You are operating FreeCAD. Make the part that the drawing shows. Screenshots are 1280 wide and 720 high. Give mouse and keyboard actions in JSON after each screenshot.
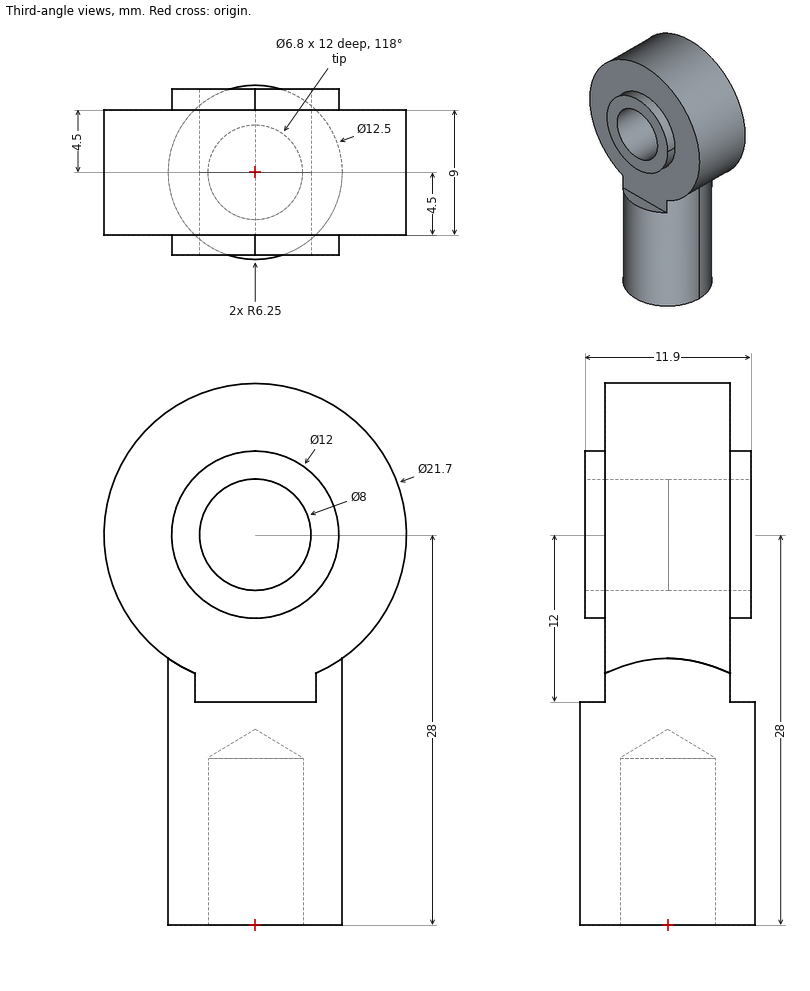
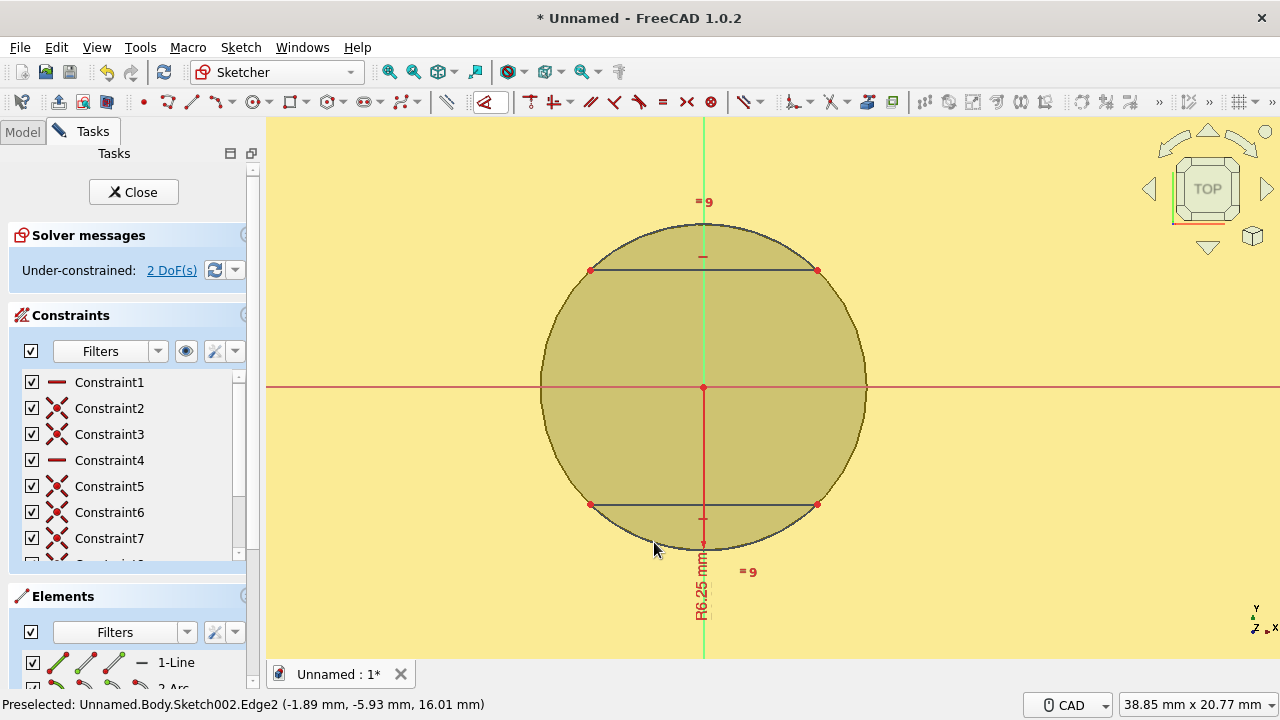
{"action": "left_click", "coordinate": [817, 505]}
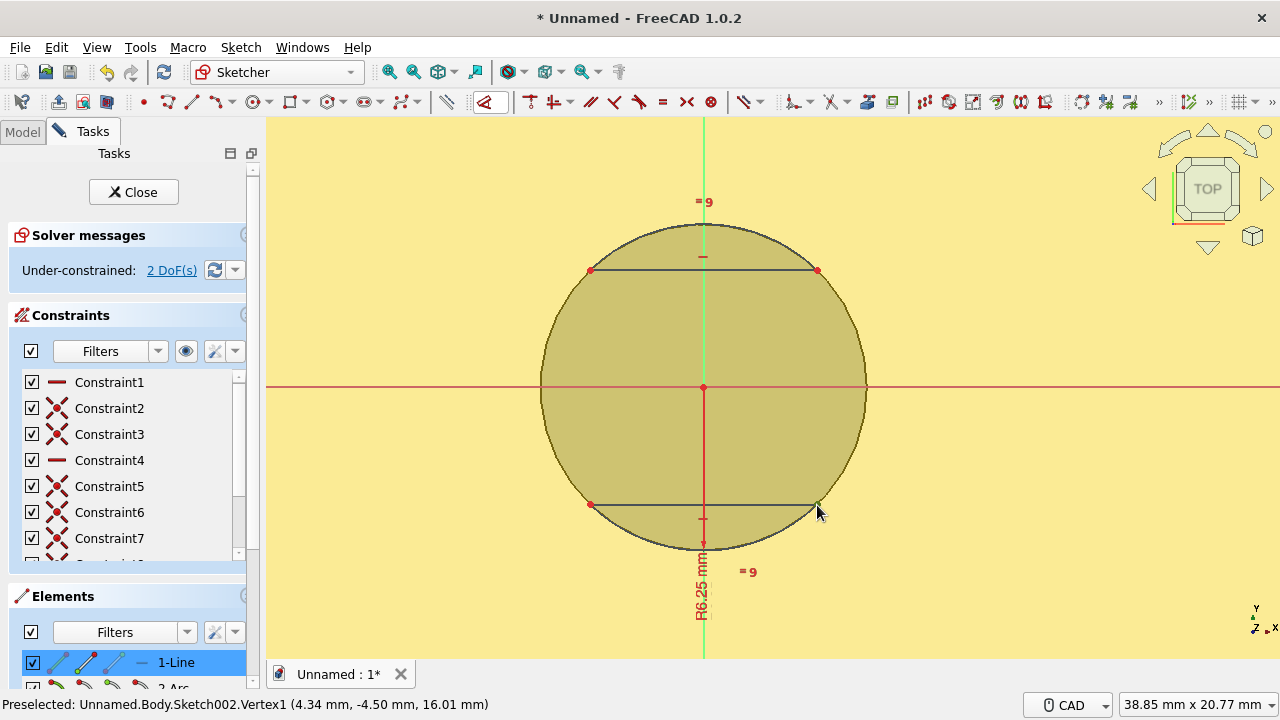
{"action": "key", "text": "i"}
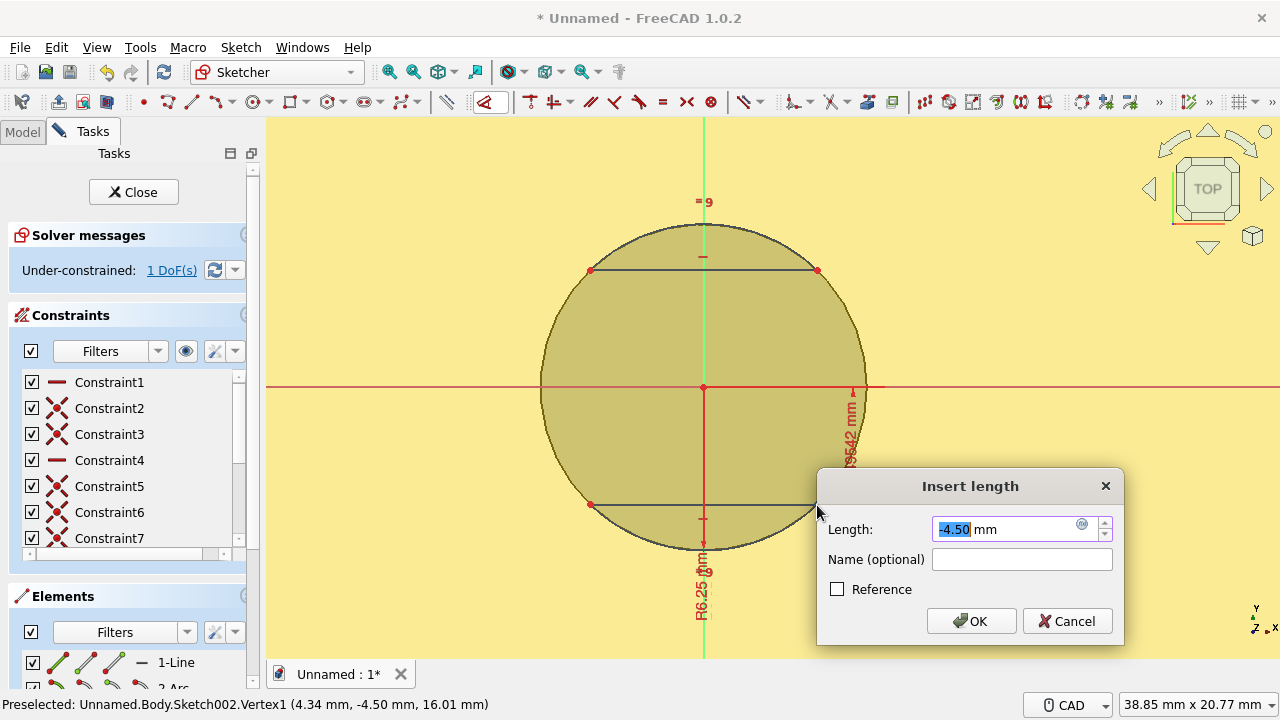
{"action": "type", "text": "-4.5"}
{"action": "key", "text": "Return"}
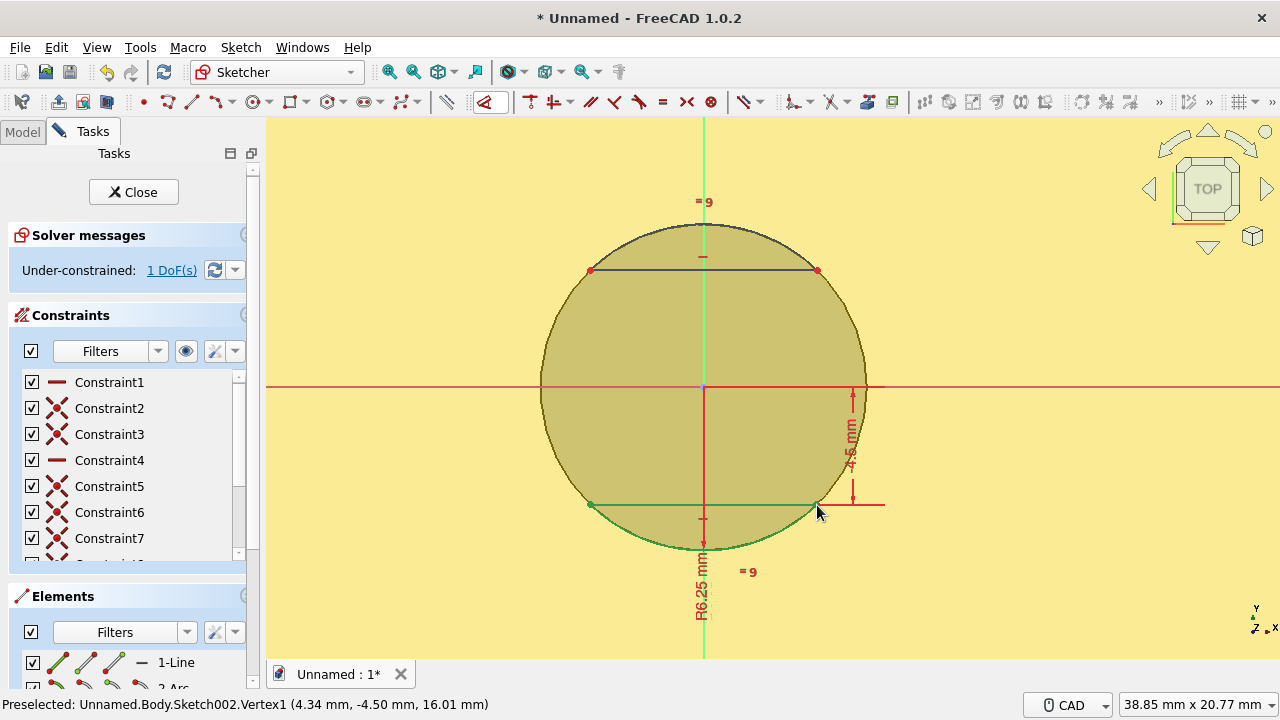
{"action": "left_click", "coordinate": [590, 270]}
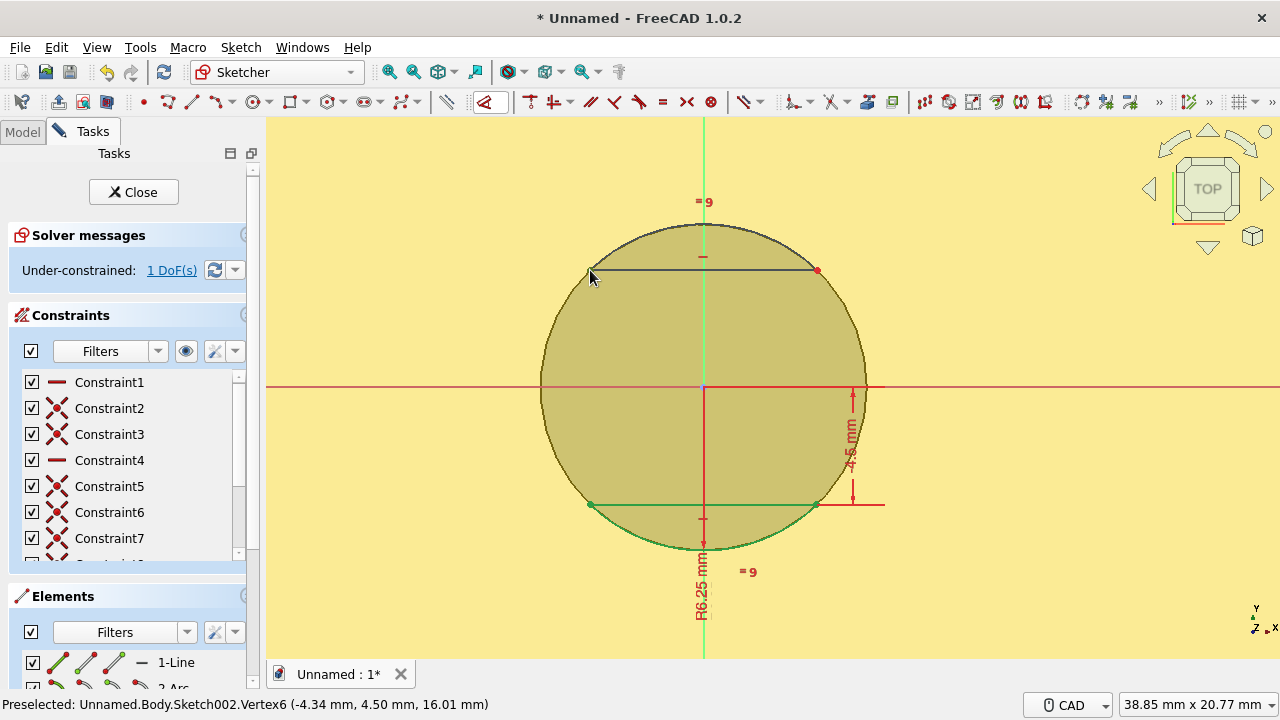
{"action": "left_click", "coordinate": [502, 102]}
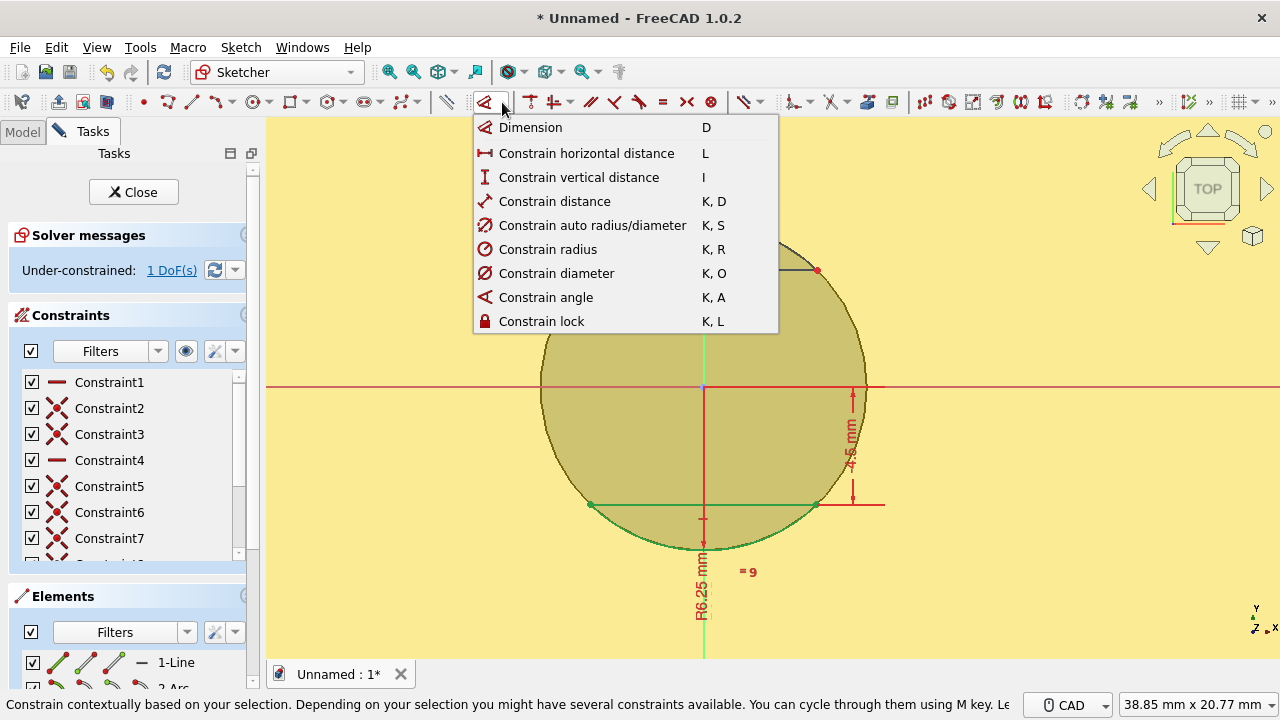
{"action": "left_click", "coordinate": [626, 177]}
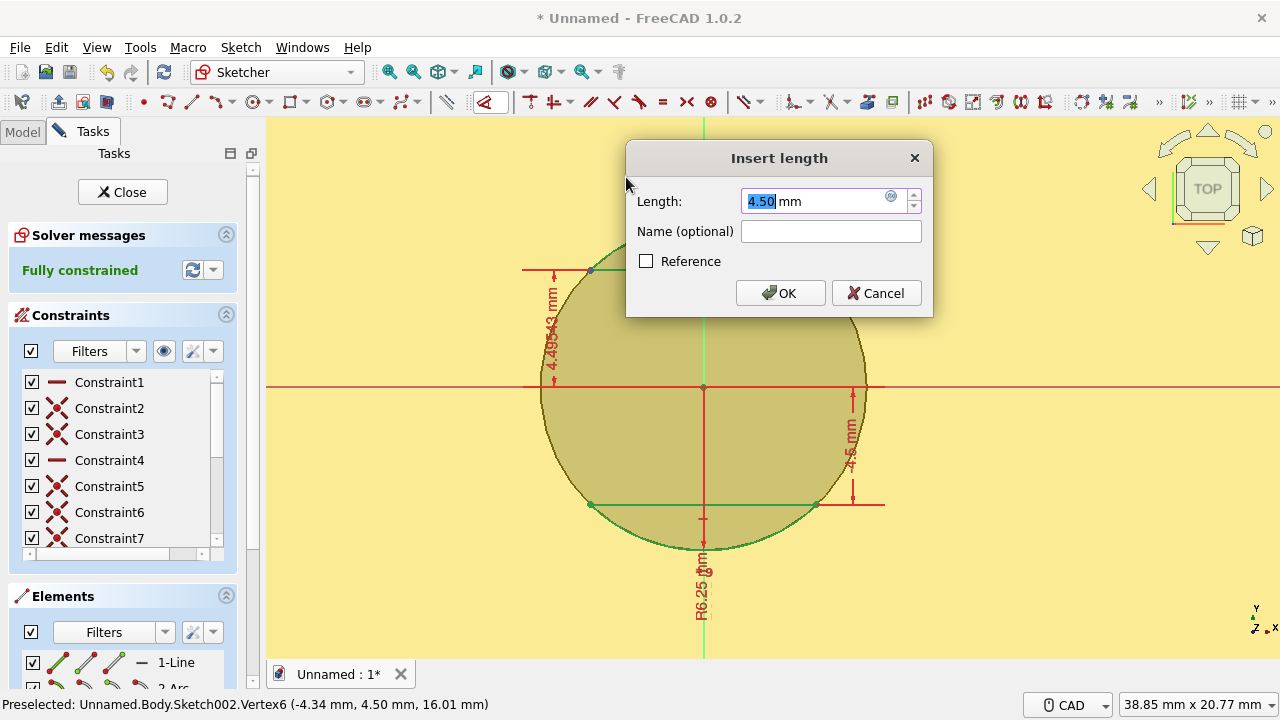
{"action": "type", "text": "4.5"}
{"action": "key", "text": "Return"}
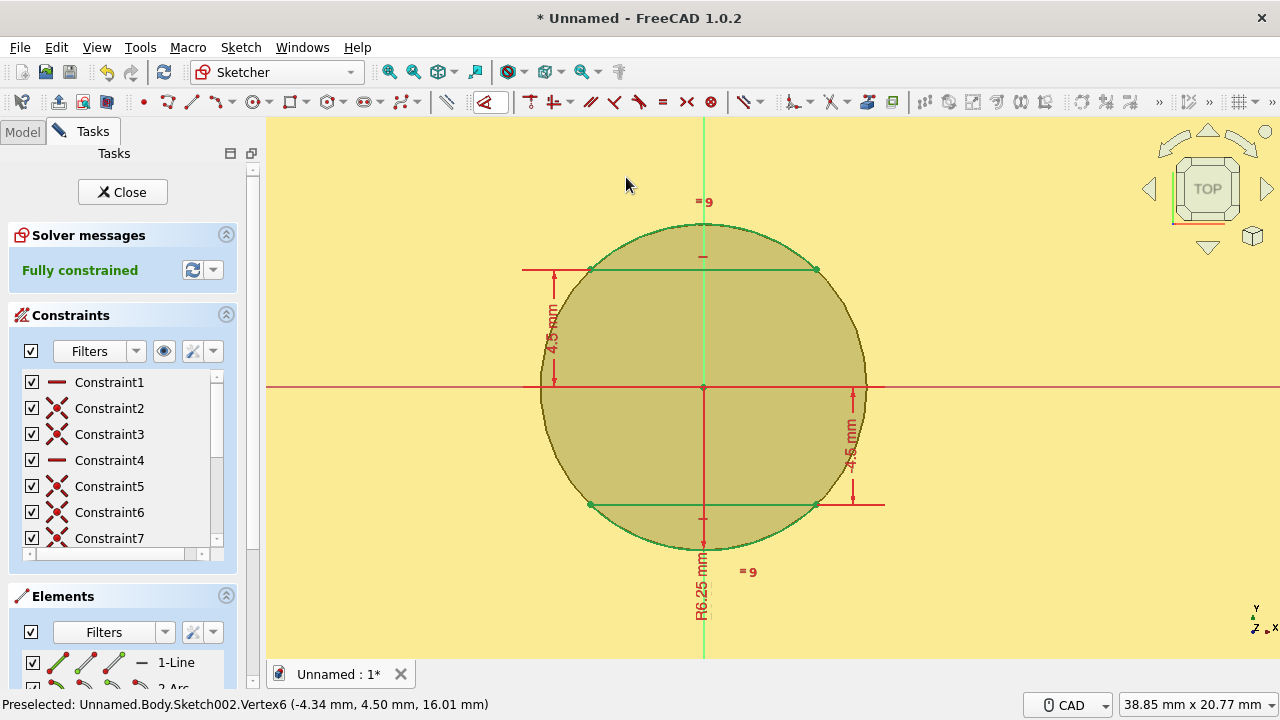
{"action": "left_click", "coordinate": [123, 192]}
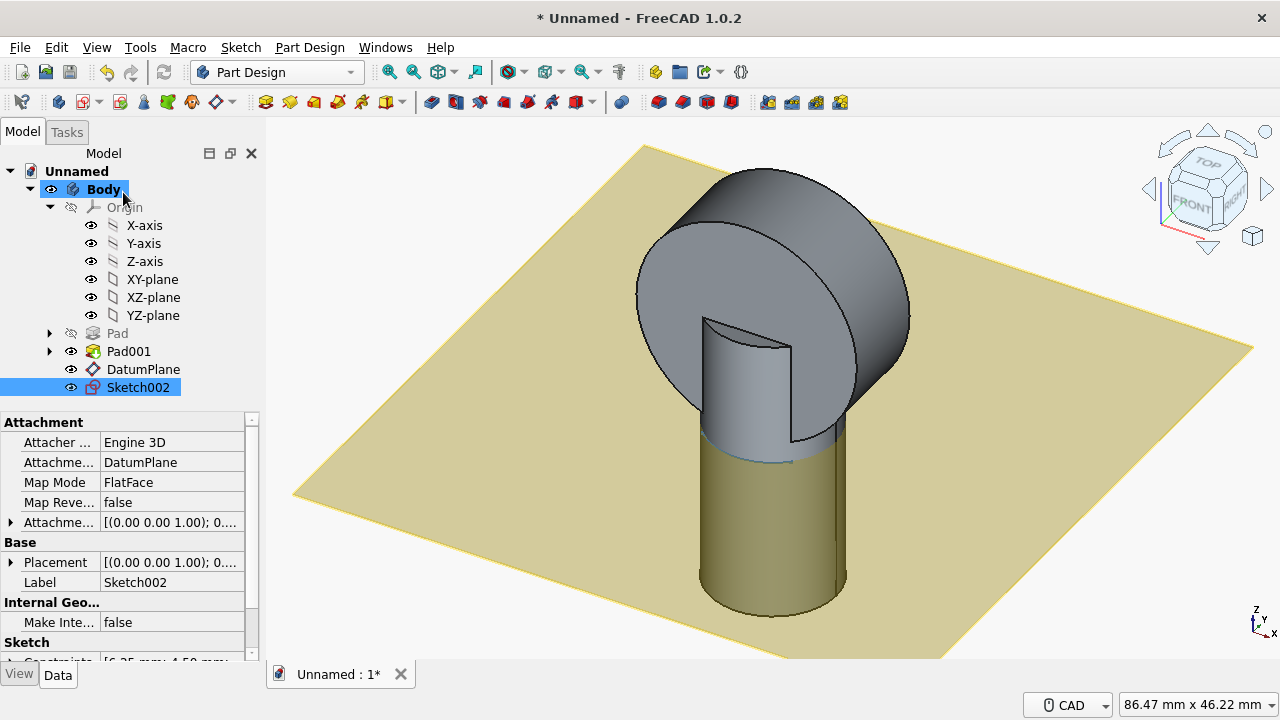
{"action": "left_click", "coordinate": [432, 102]}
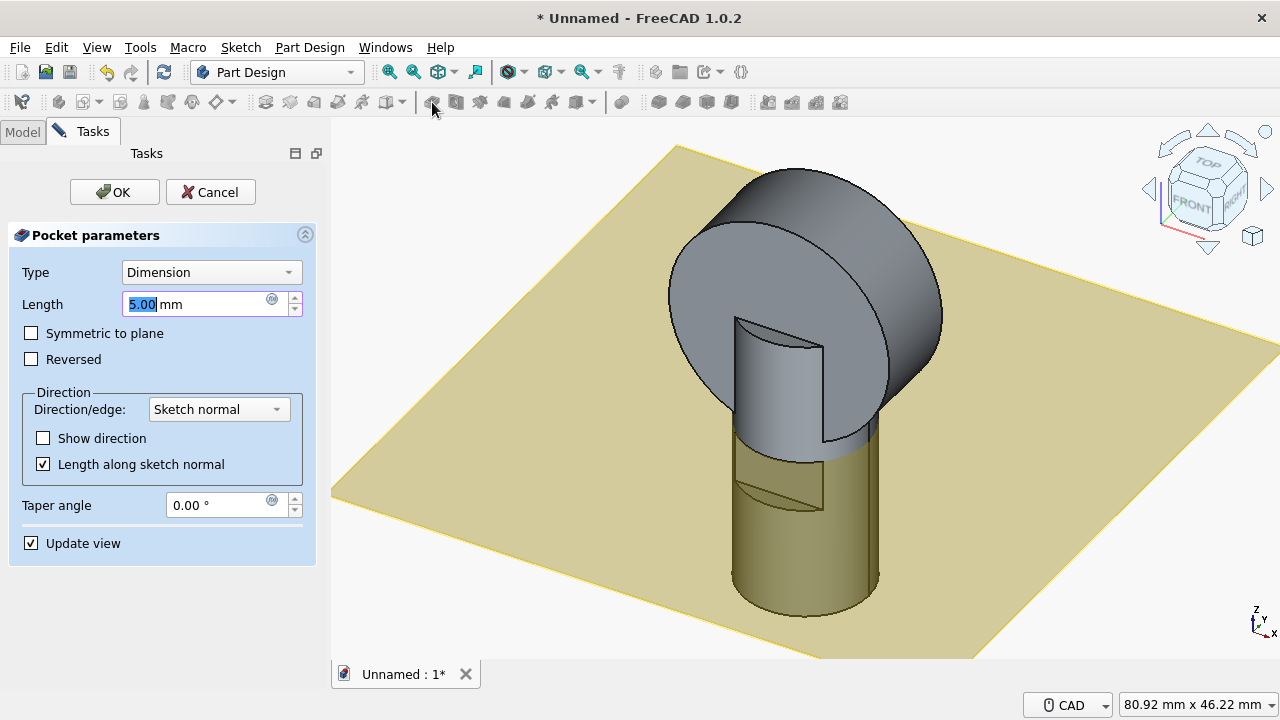
{"action": "type", "text": "12"}
{"action": "key", "text": "Tab"}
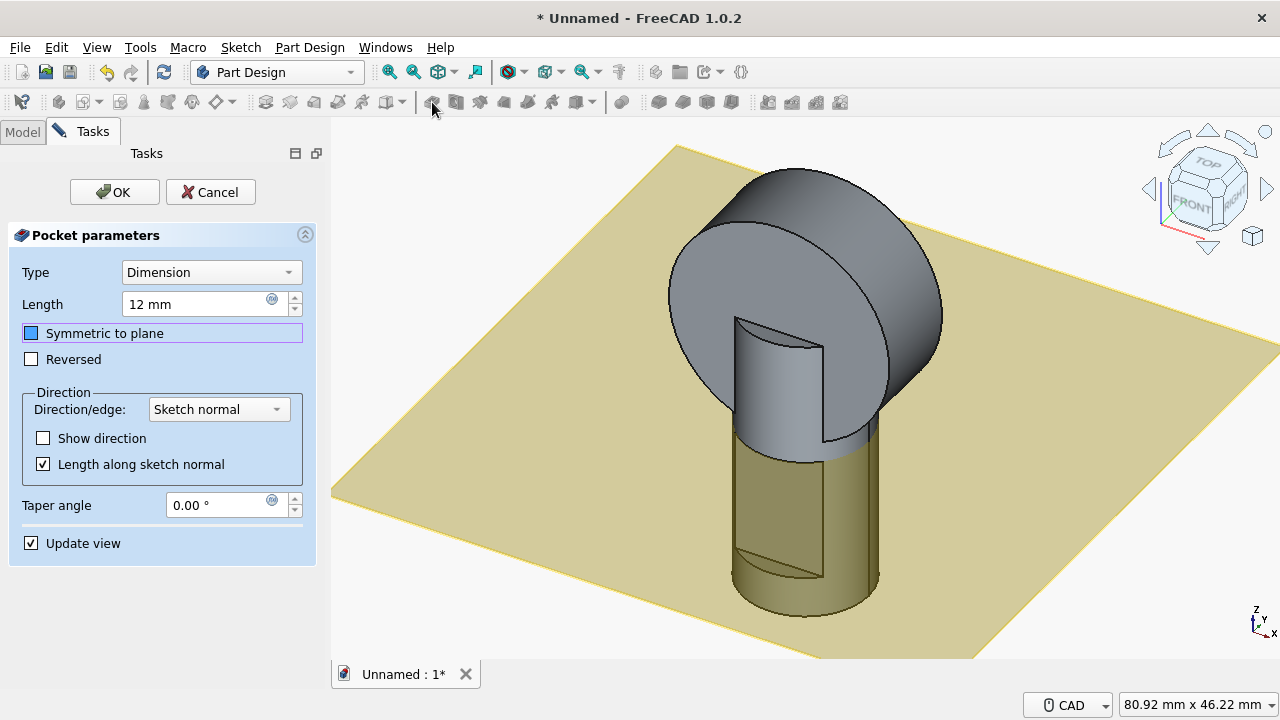
{"action": "left_click", "coordinate": [30, 359]}